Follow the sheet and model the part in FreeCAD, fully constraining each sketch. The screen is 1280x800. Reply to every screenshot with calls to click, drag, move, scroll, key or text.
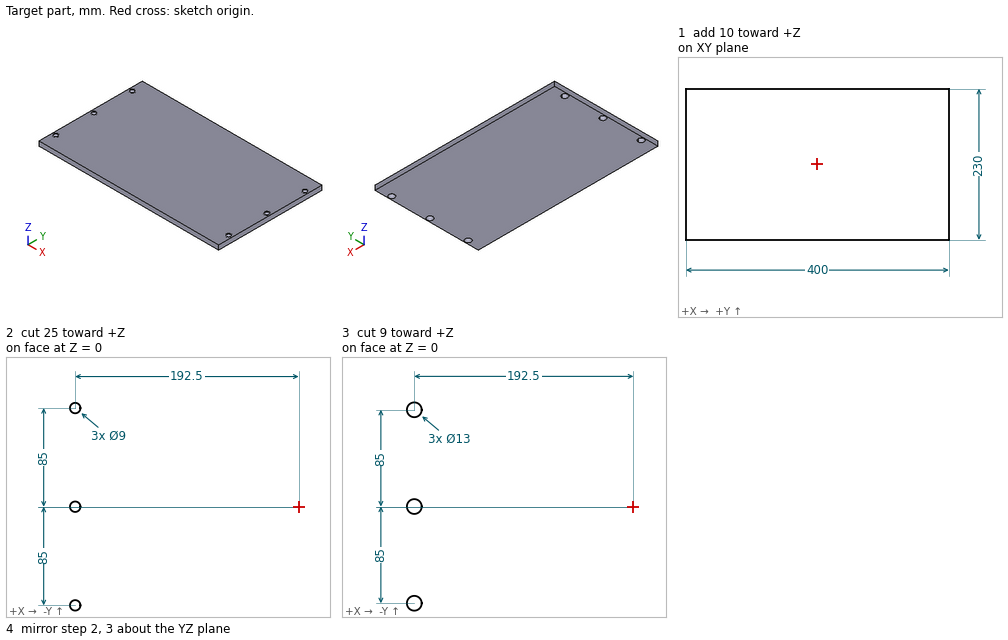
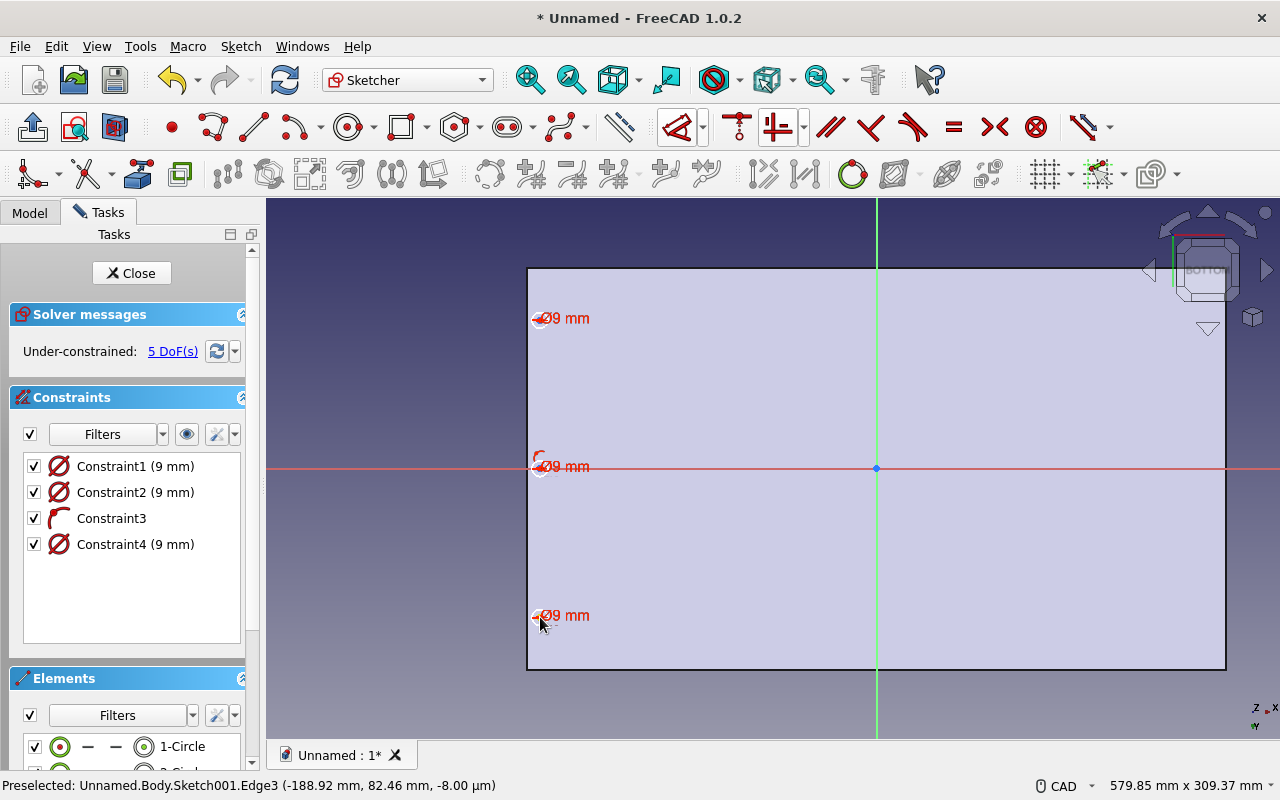
click(540, 320)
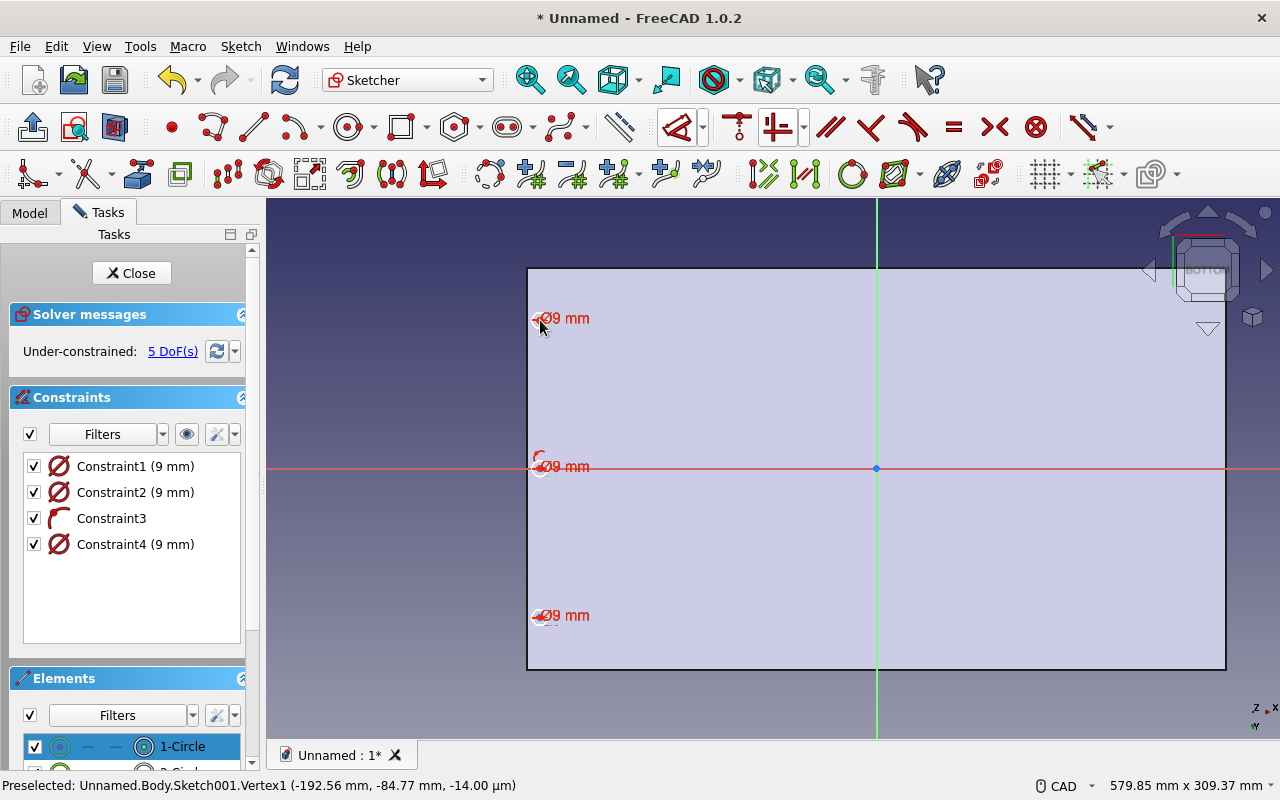
click(540, 469)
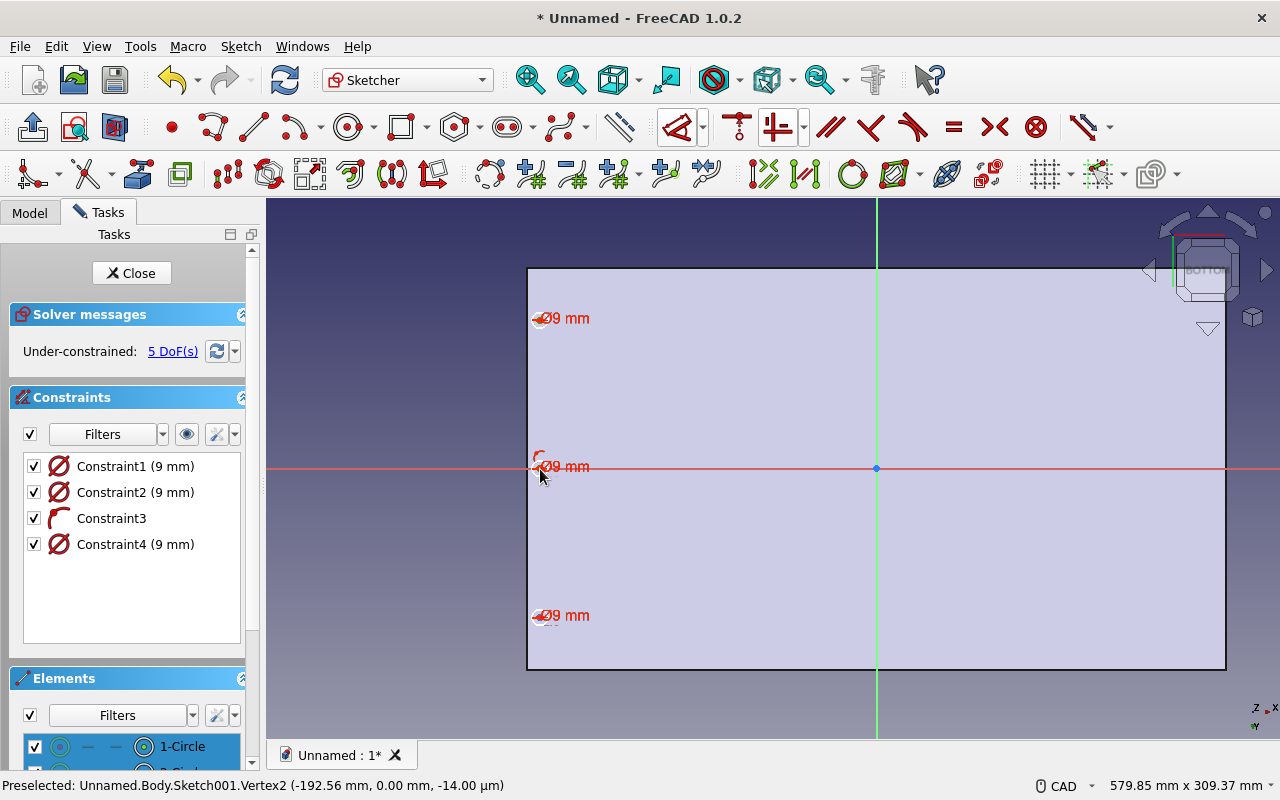
click(804, 128)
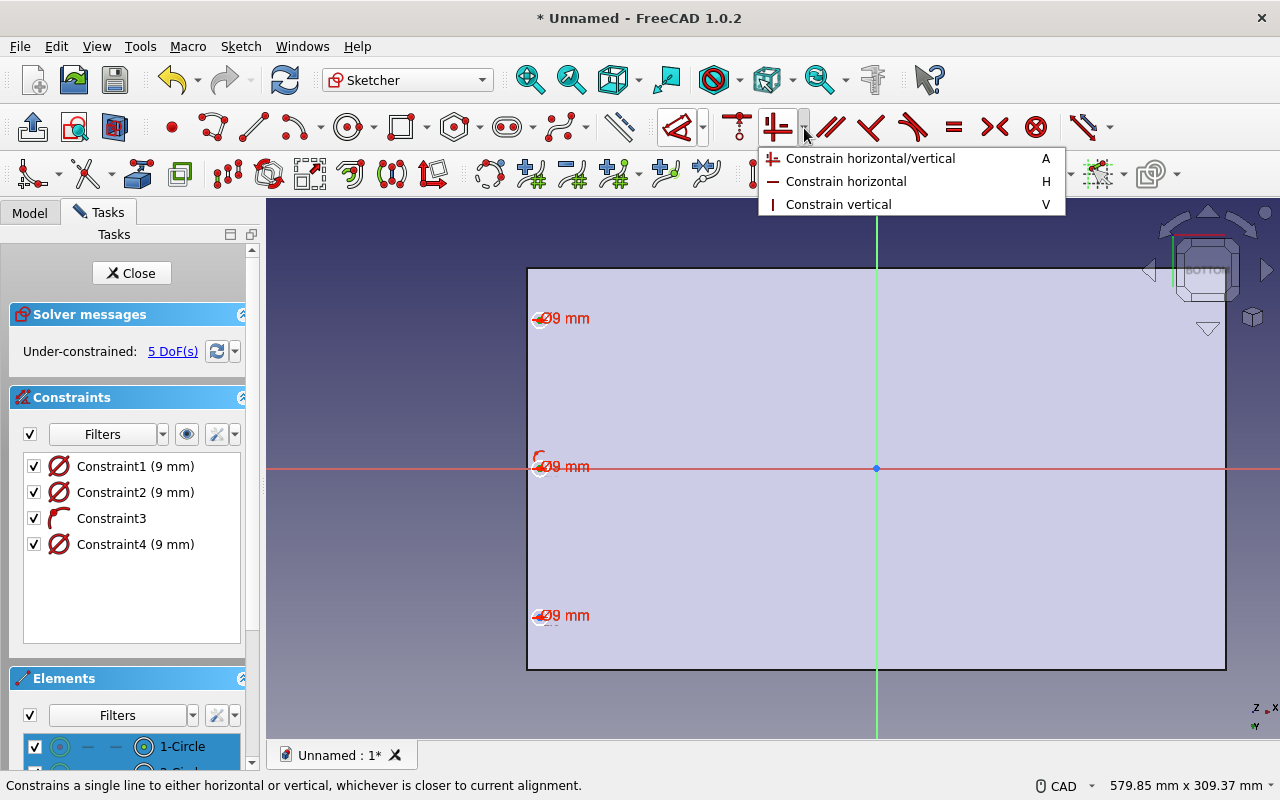
click(912, 204)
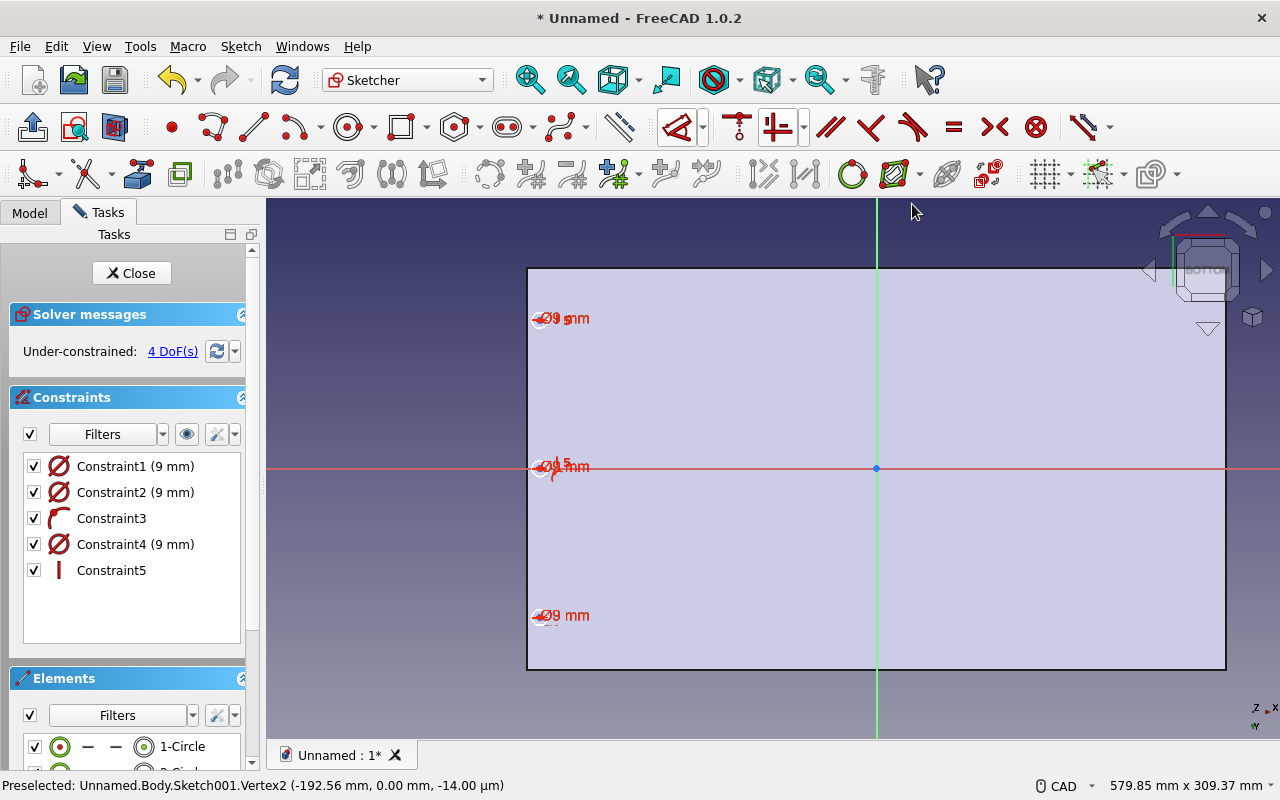
click(540, 469)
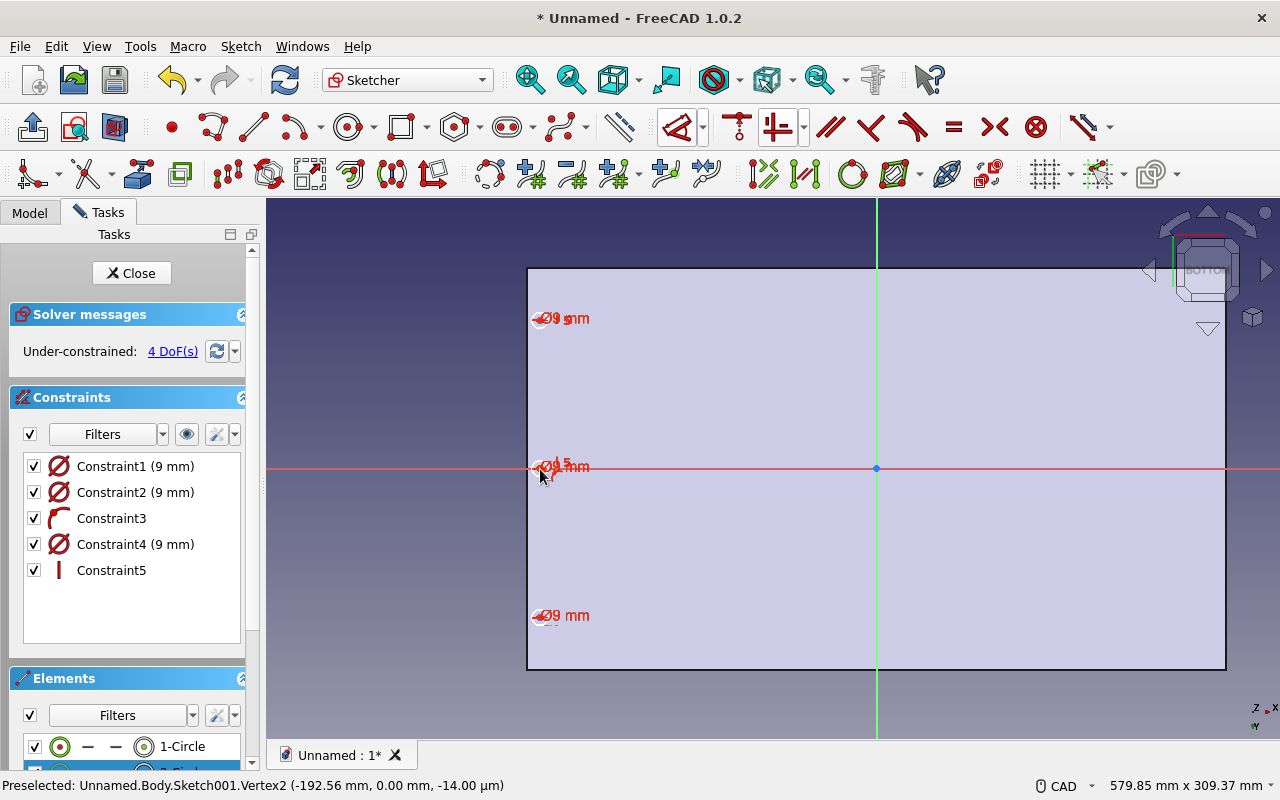
click(540, 618)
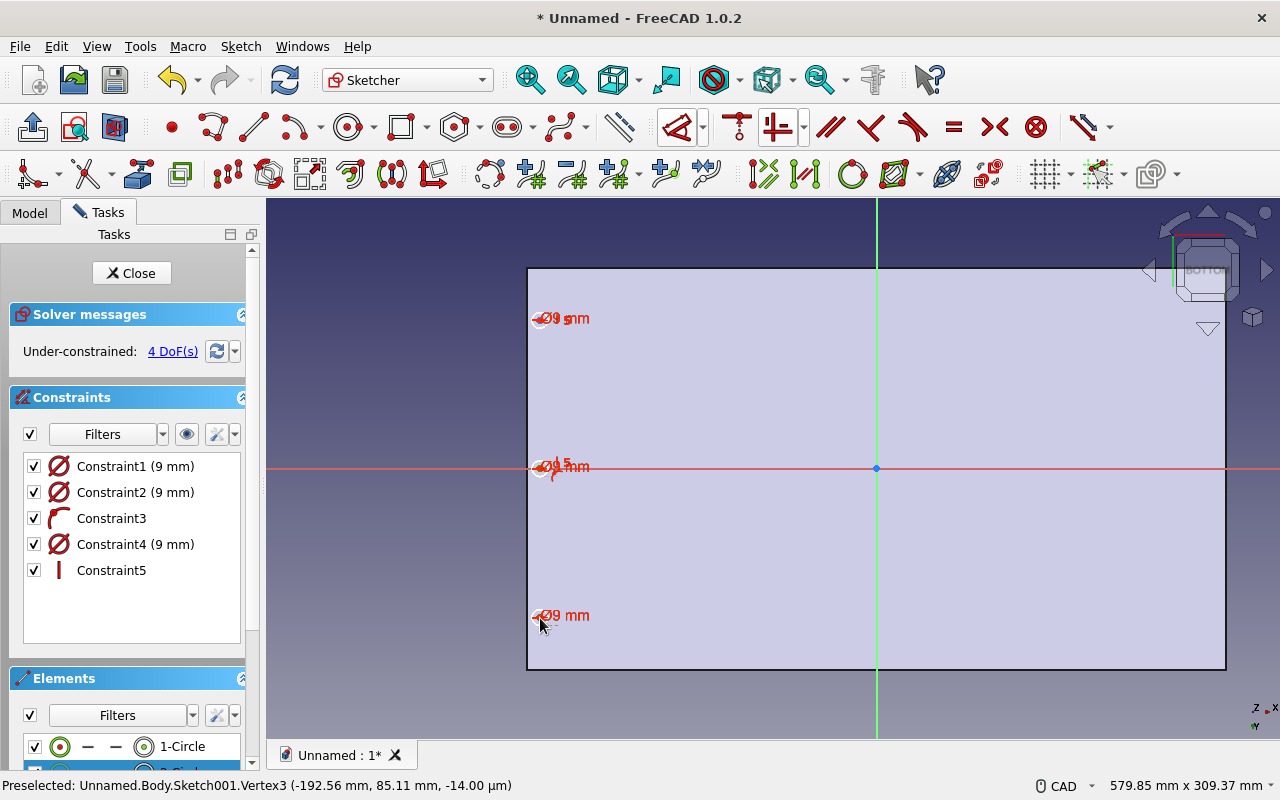
click(804, 128)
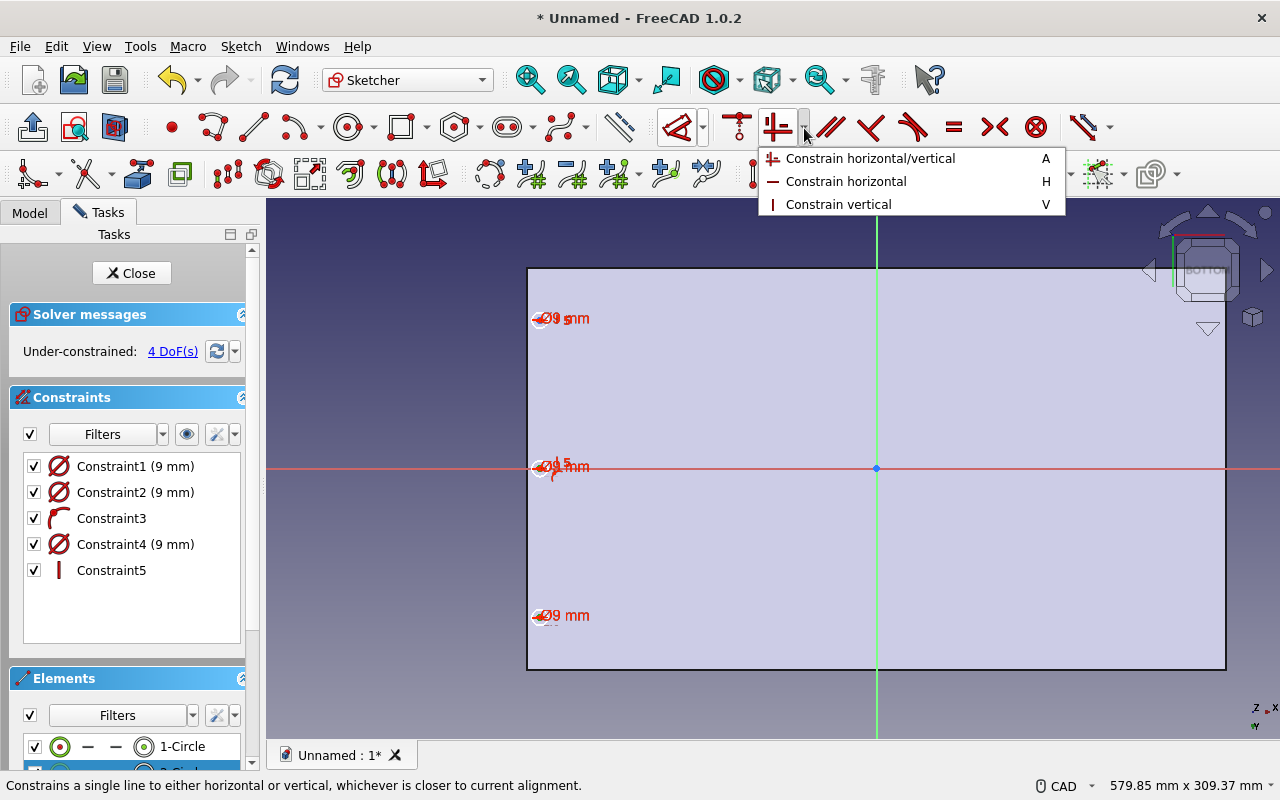
click(912, 204)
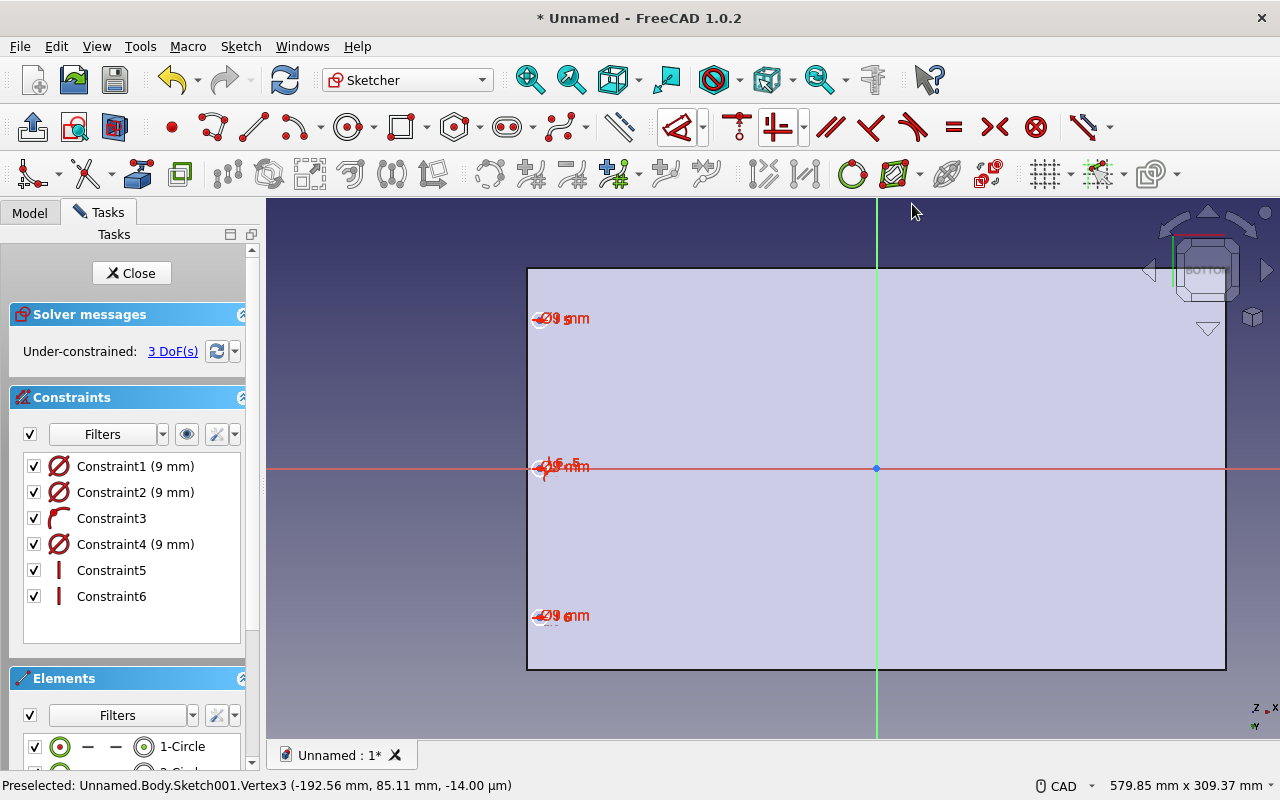
click(676, 128)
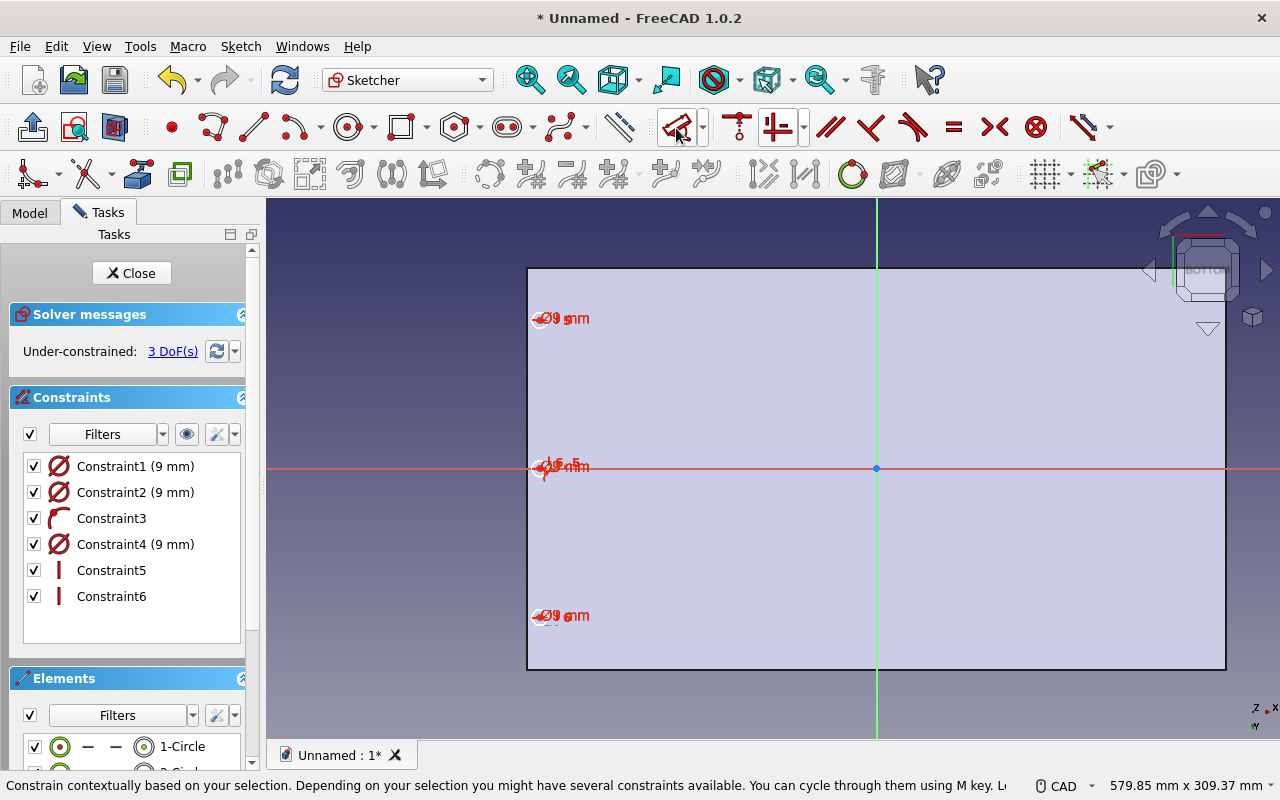
click(540, 320)
click(911, 395)